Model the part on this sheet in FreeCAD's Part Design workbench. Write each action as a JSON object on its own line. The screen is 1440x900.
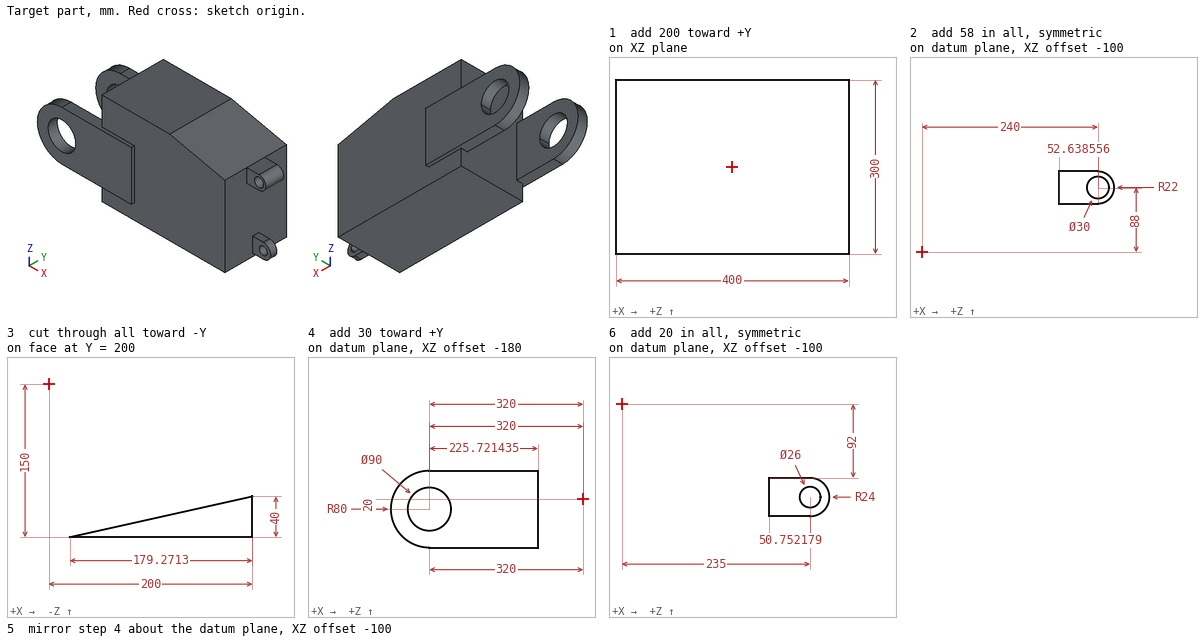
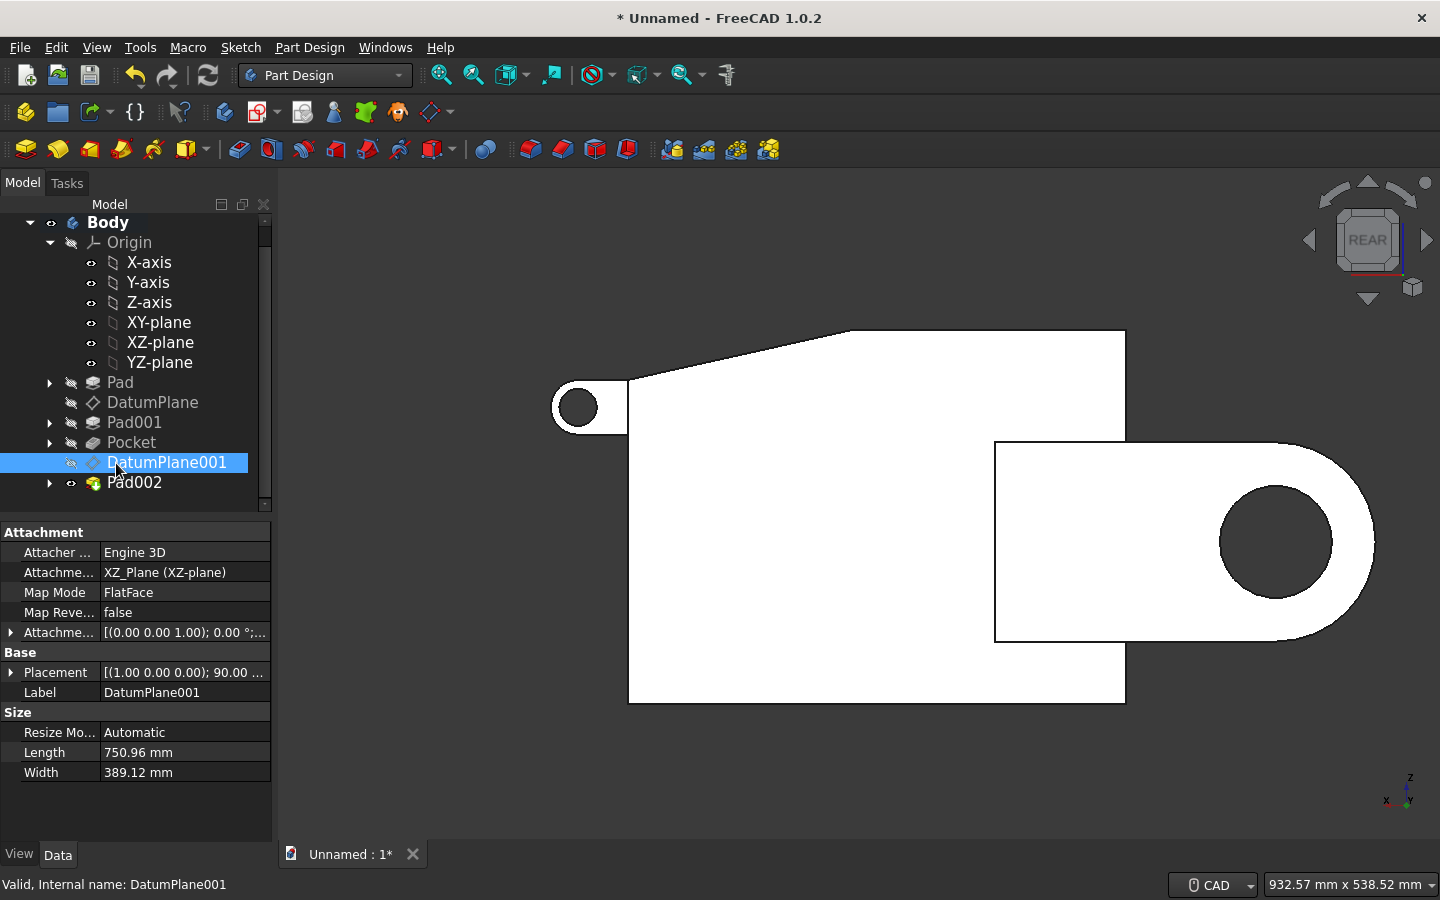
{"action": "left_click", "coordinate": [136, 343]}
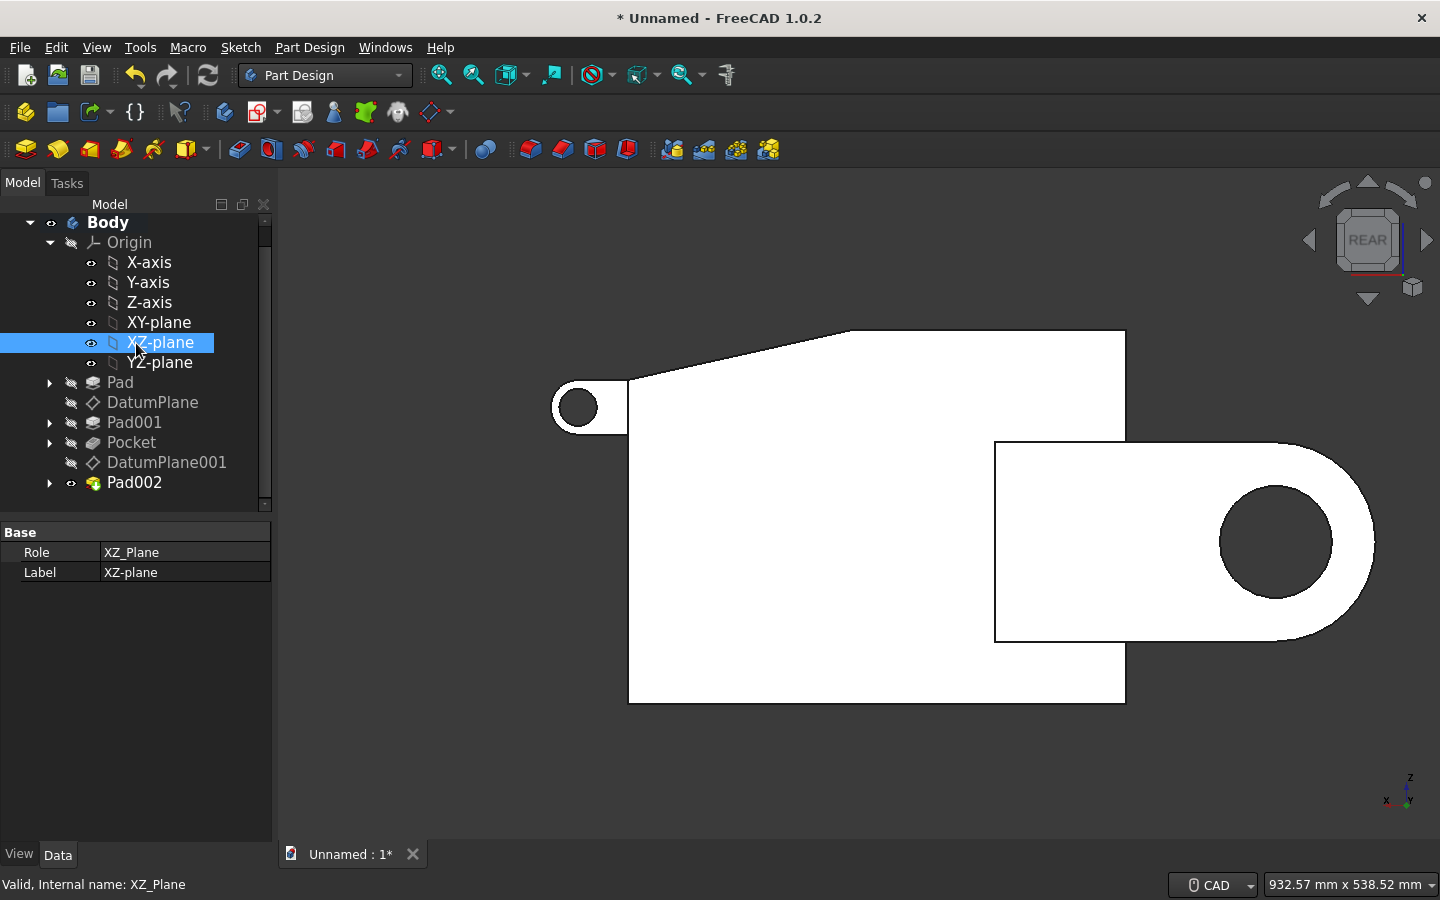
{"action": "left_click", "coordinate": [430, 112]}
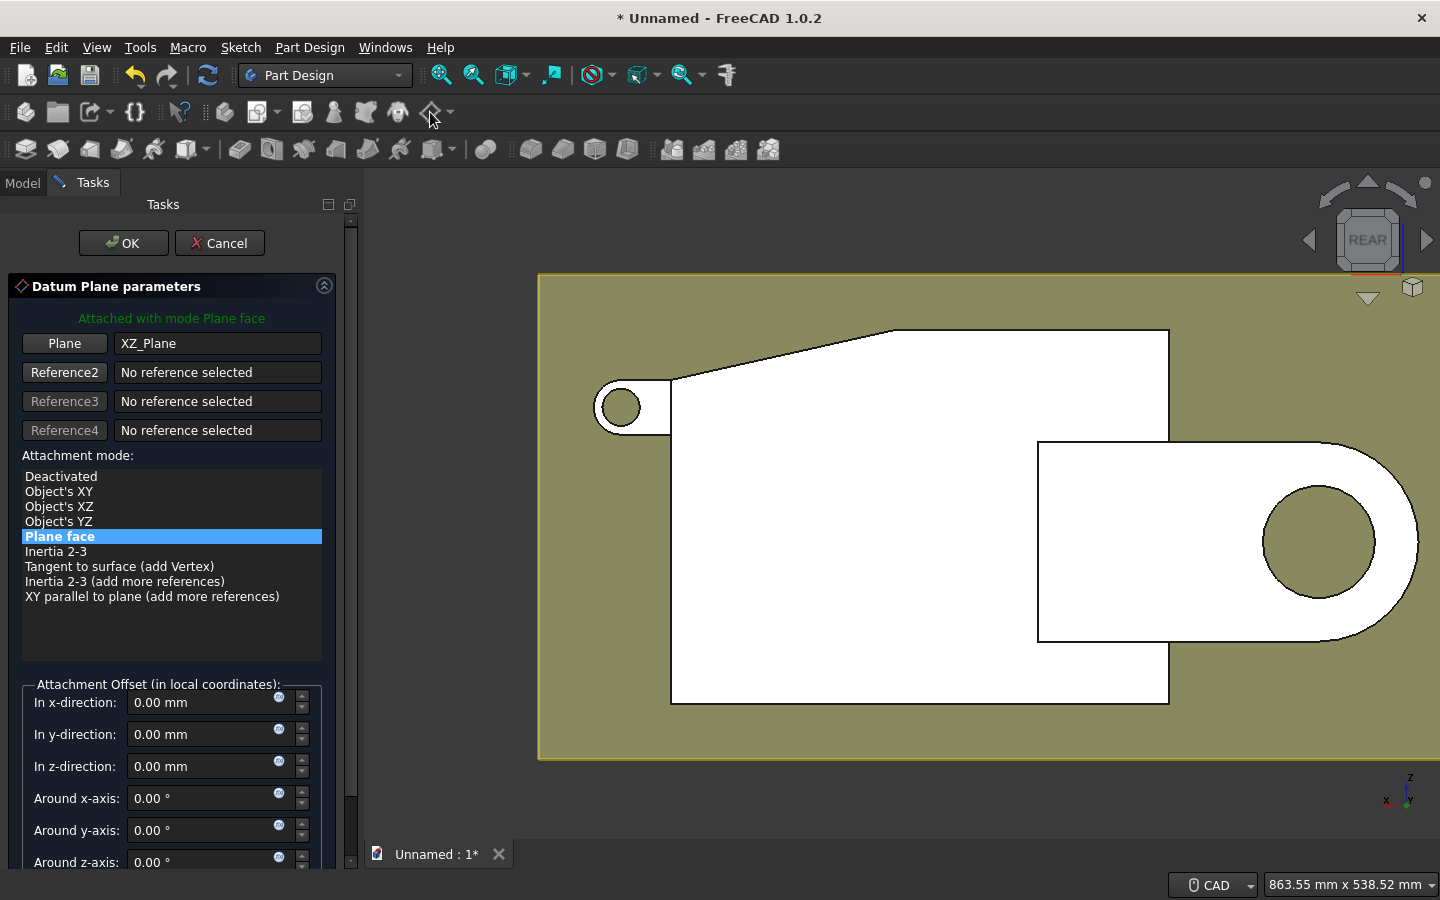
{"action": "triple_click", "coordinate": [210, 766]}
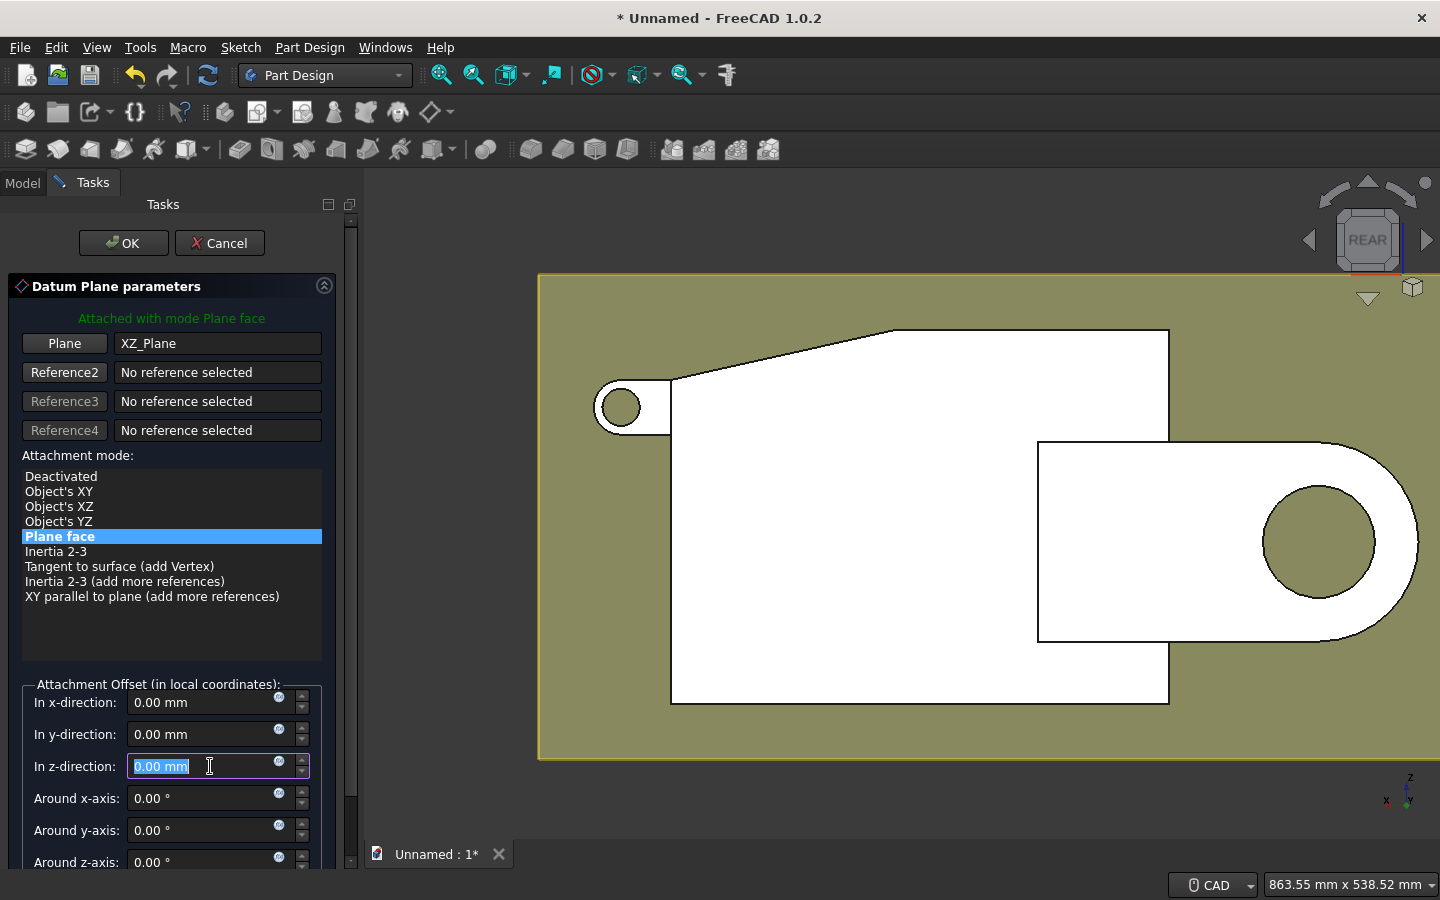
{"action": "type", "text": "-100"}
{"action": "key", "text": "Tab"}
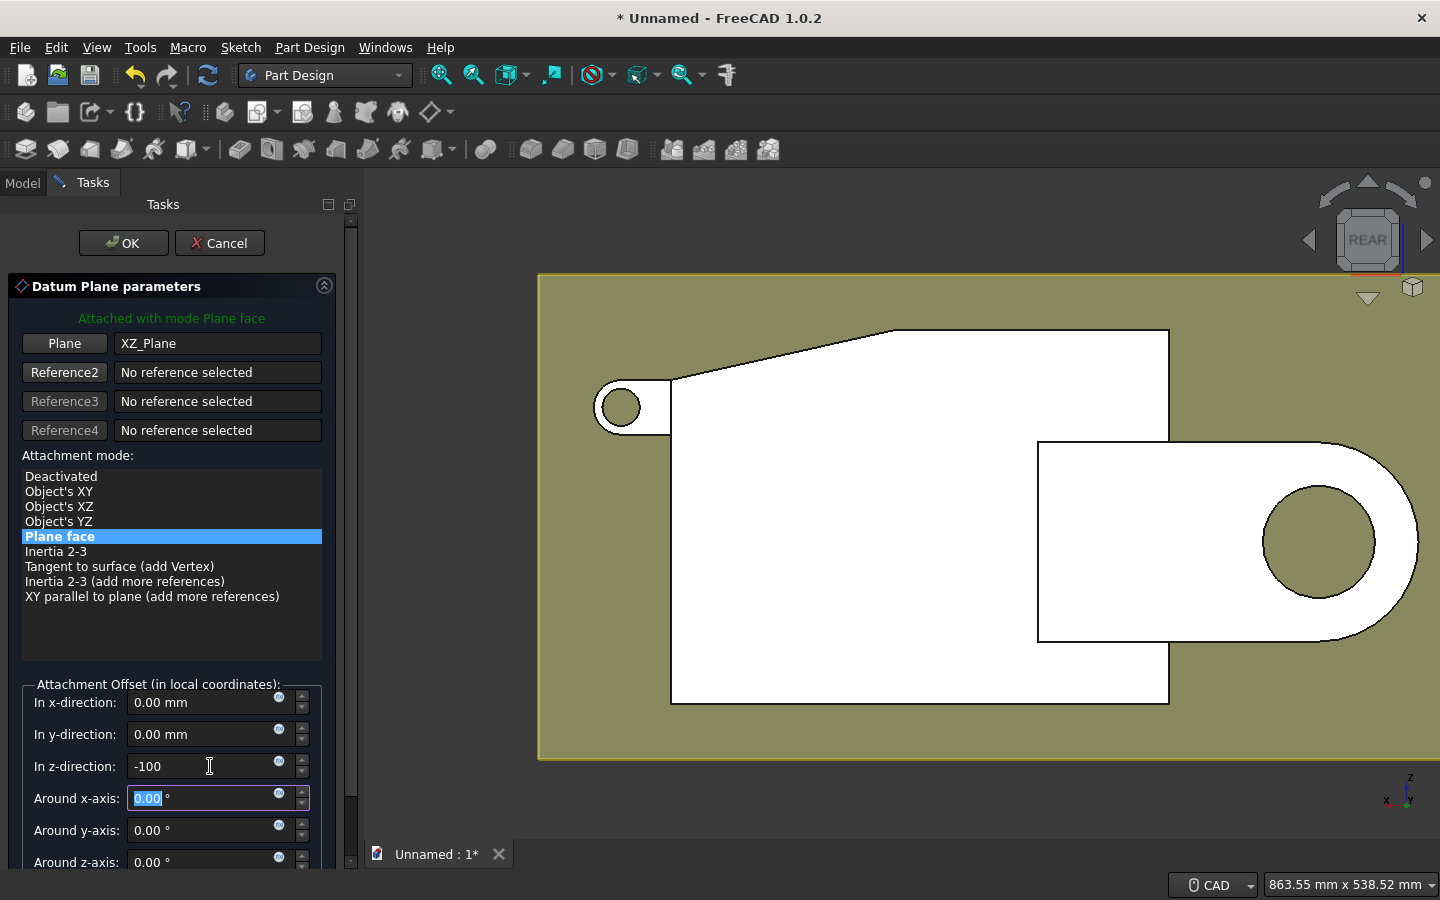
{"action": "left_click", "coordinate": [124, 243]}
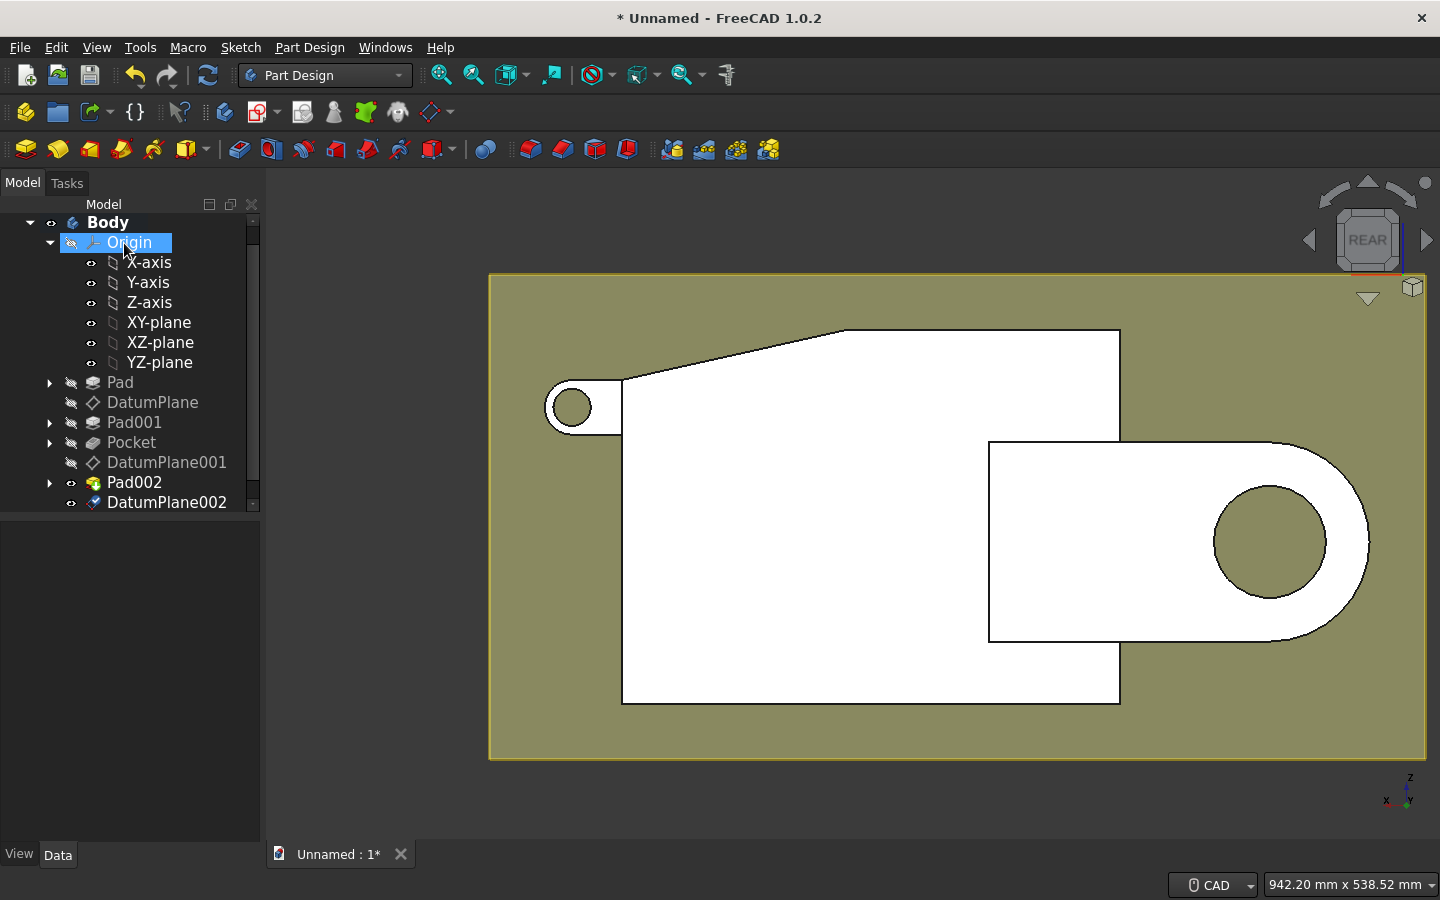
{"action": "left_click", "coordinate": [116, 483]}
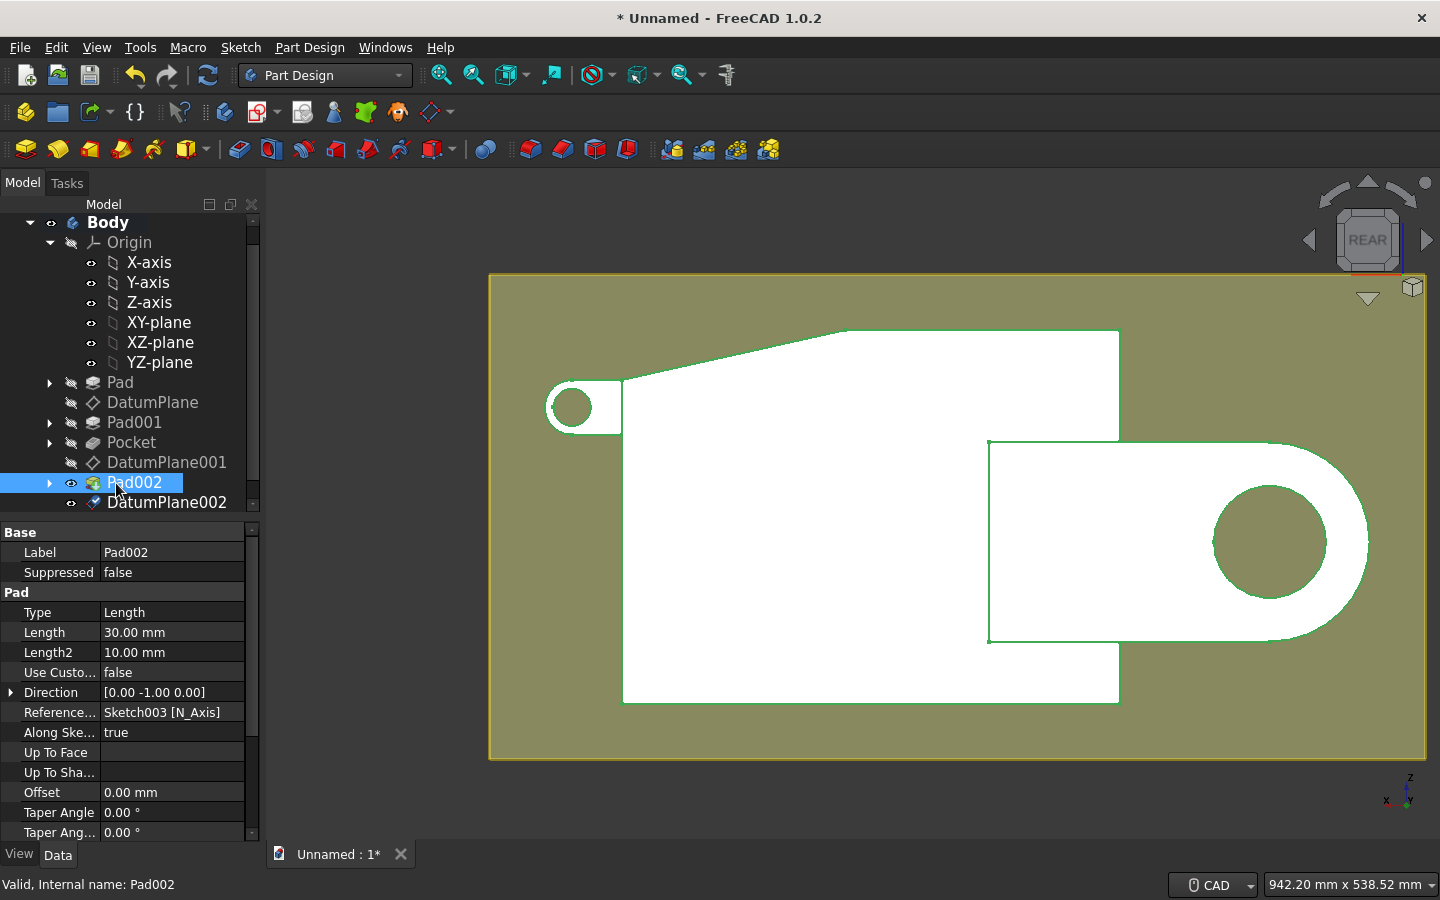
{"action": "left_click", "coordinate": [672, 150]}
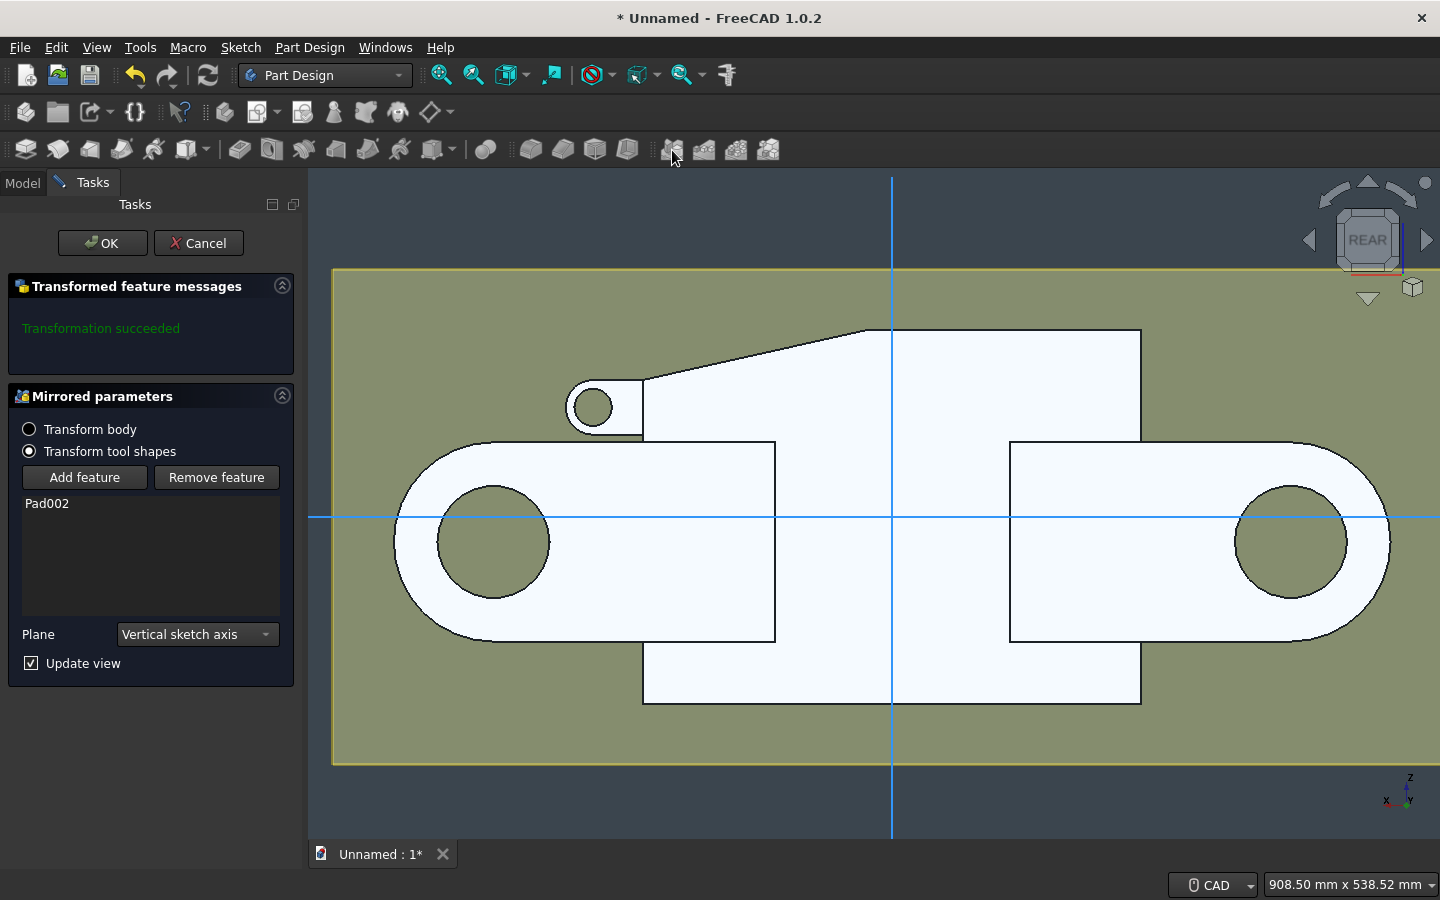
{"action": "left_click", "coordinate": [198, 634]}